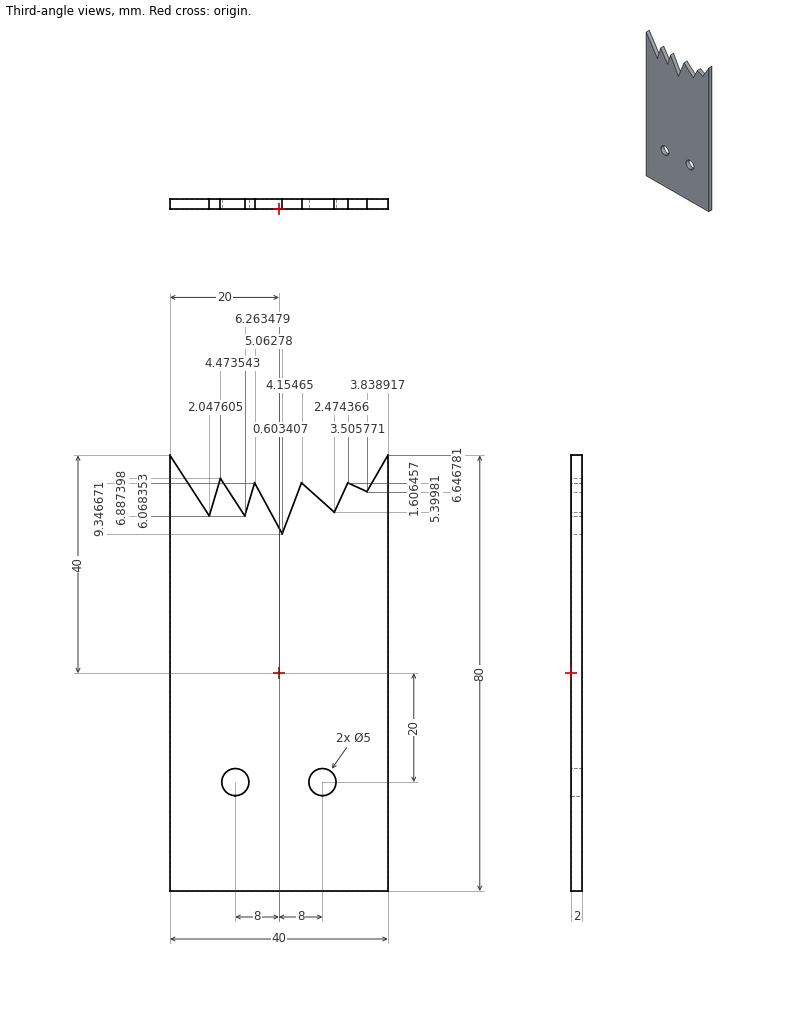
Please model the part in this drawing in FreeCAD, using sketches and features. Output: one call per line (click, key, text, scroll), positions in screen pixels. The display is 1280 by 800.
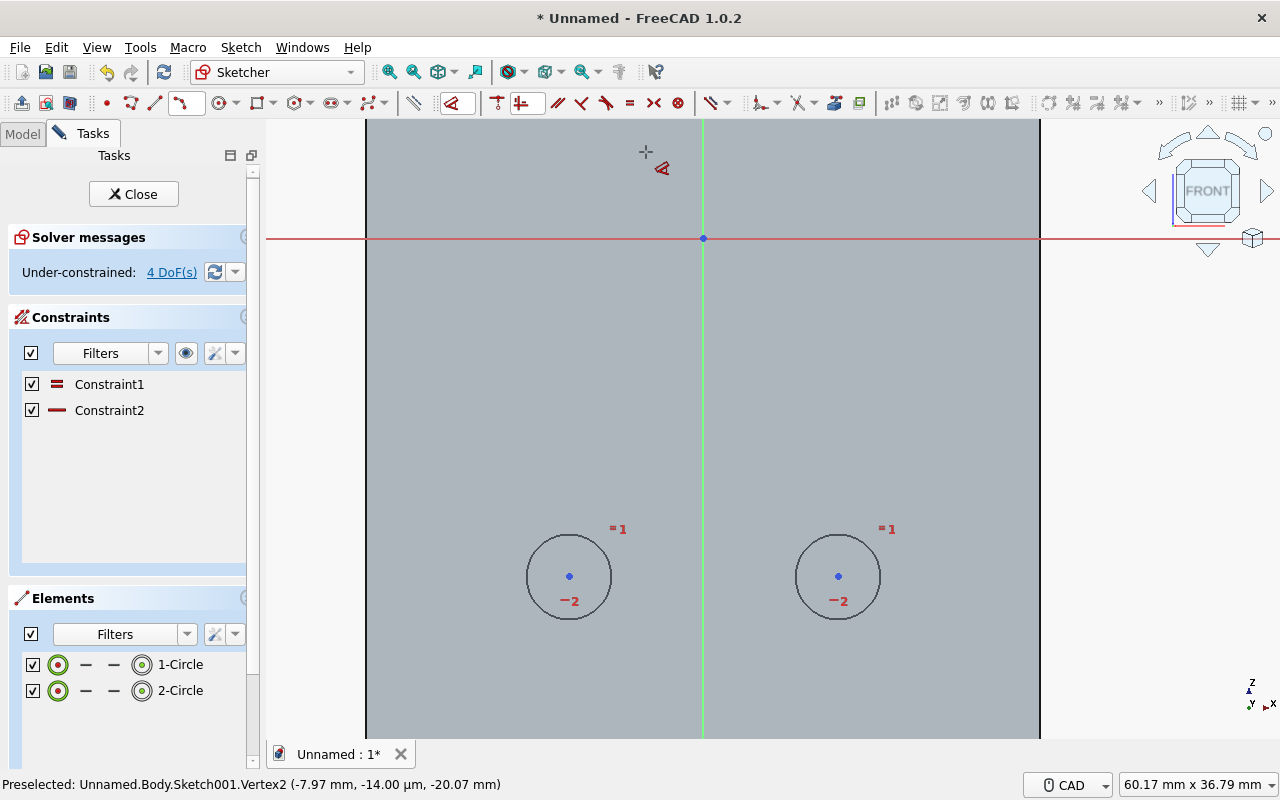
click(868, 547)
click(891, 524)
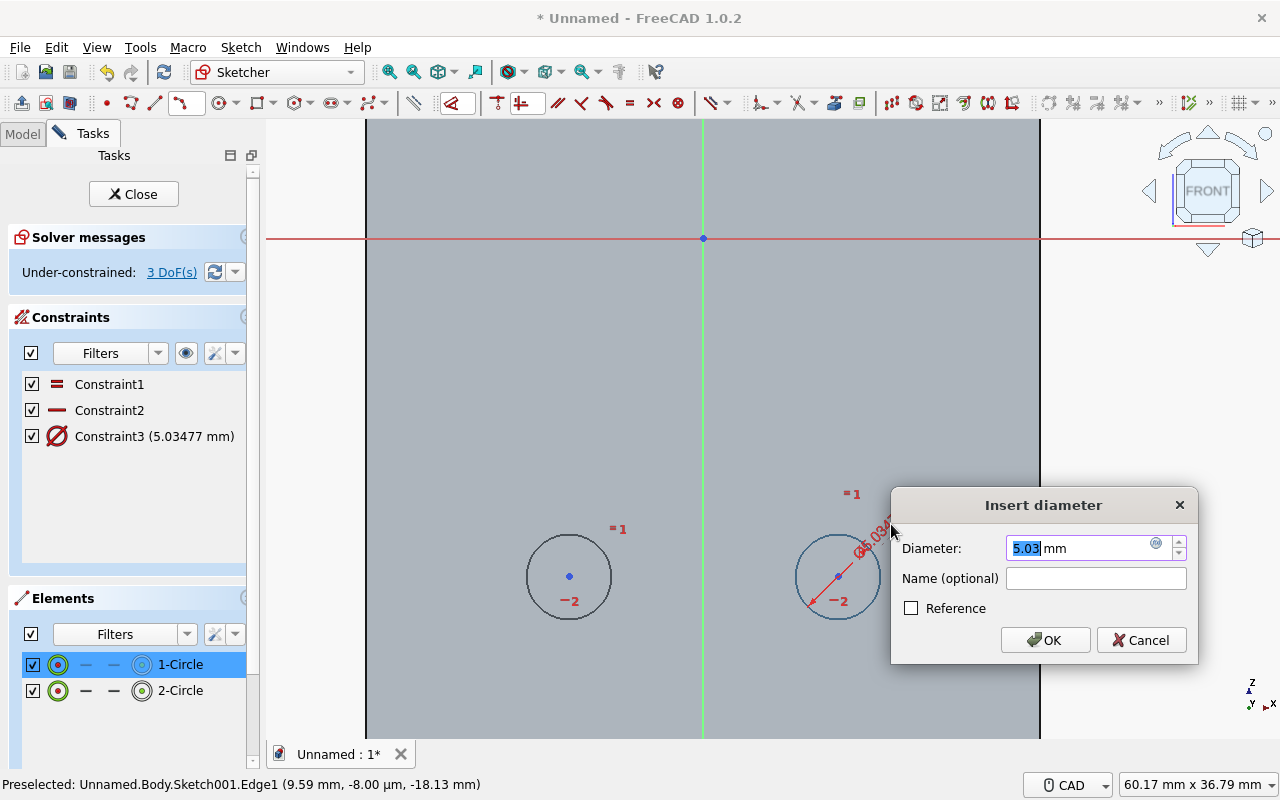
text(5)
key(Return)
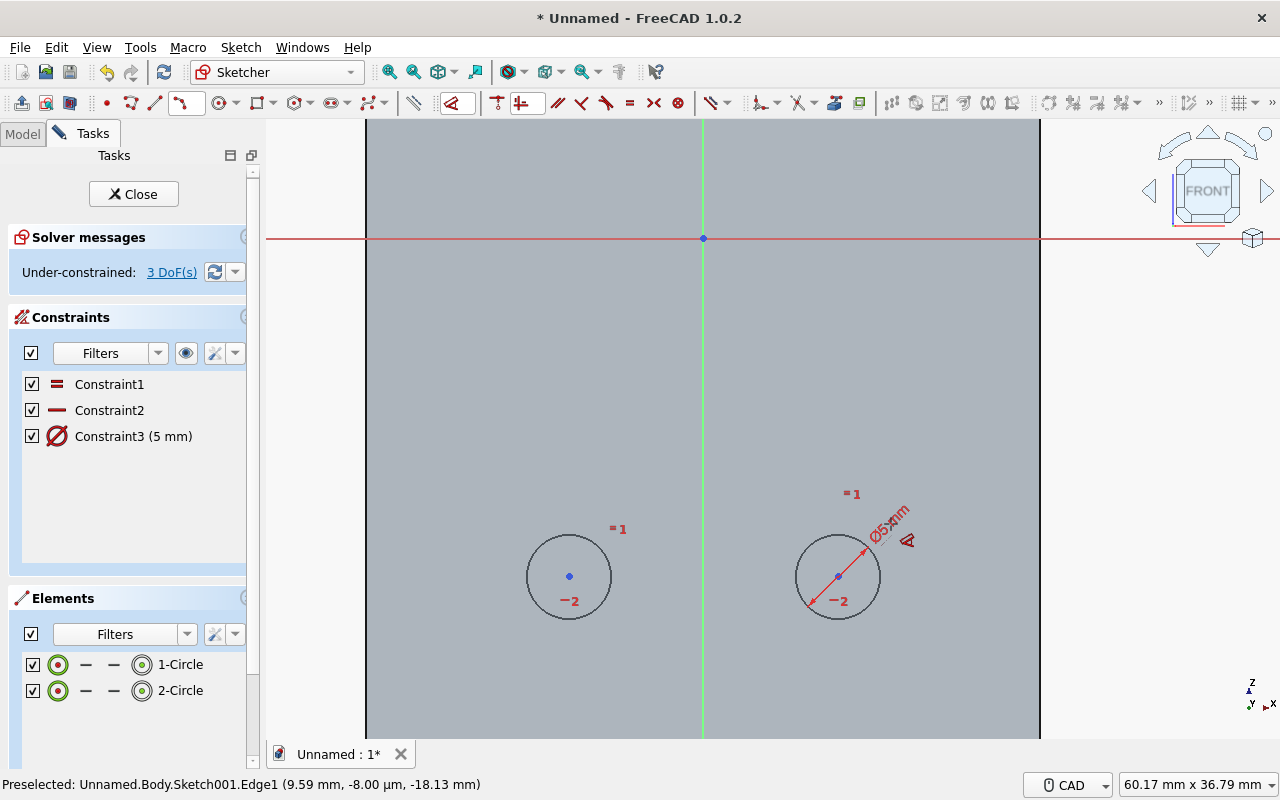
click(838, 577)
click(771, 205)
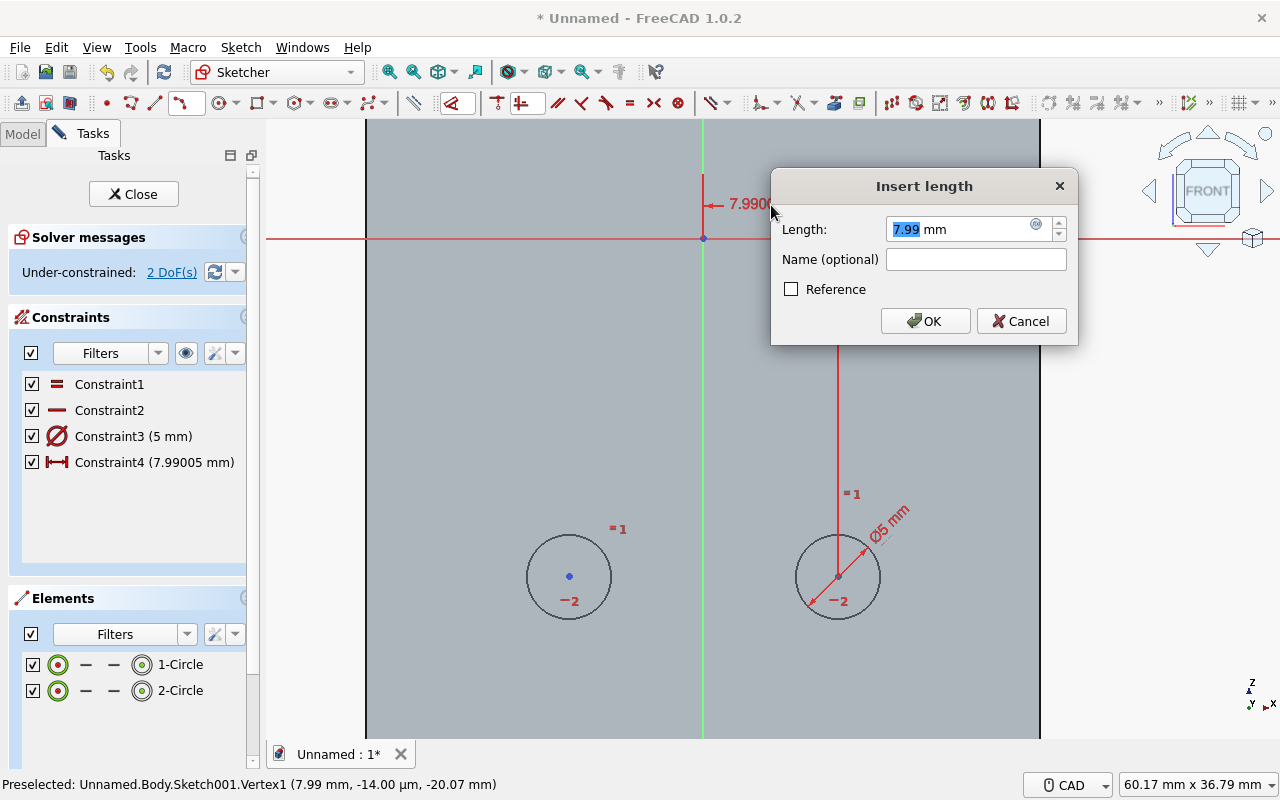
text(8)
key(Return)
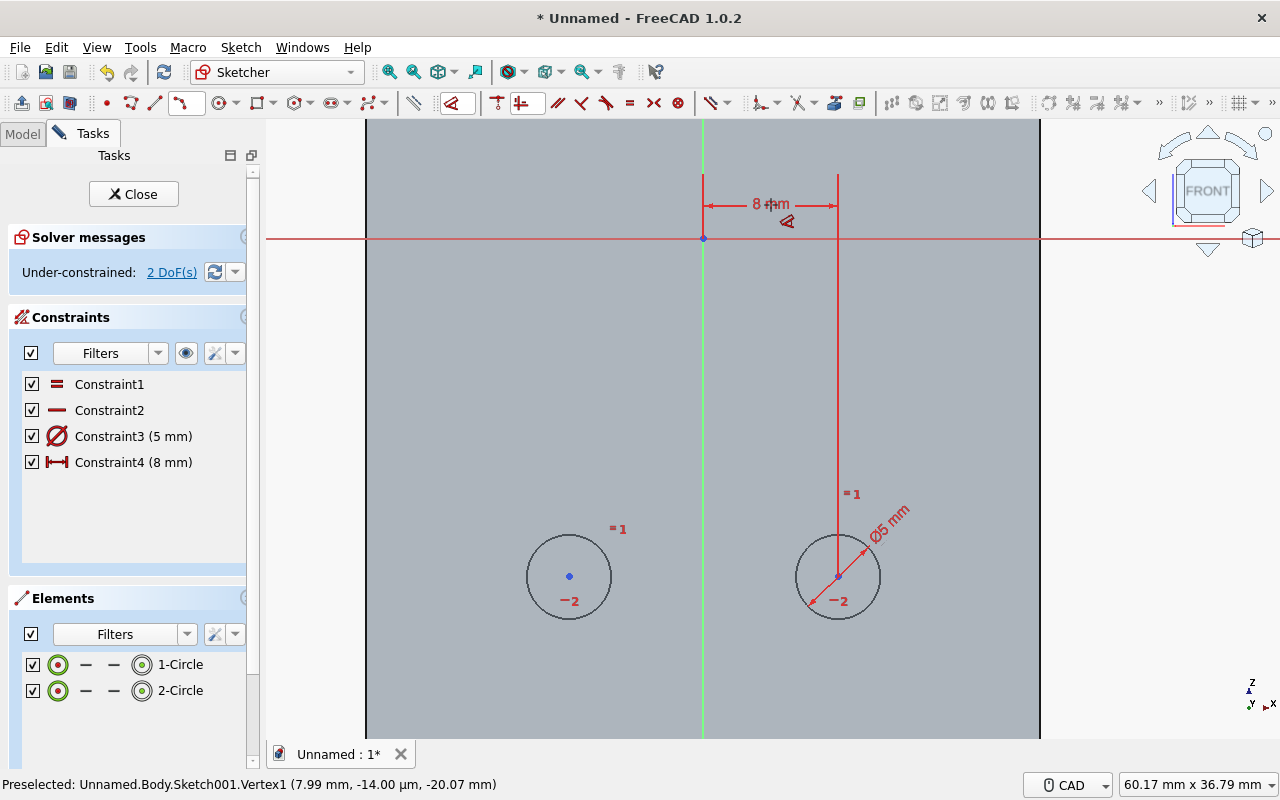
click(569, 577)
click(636, 205)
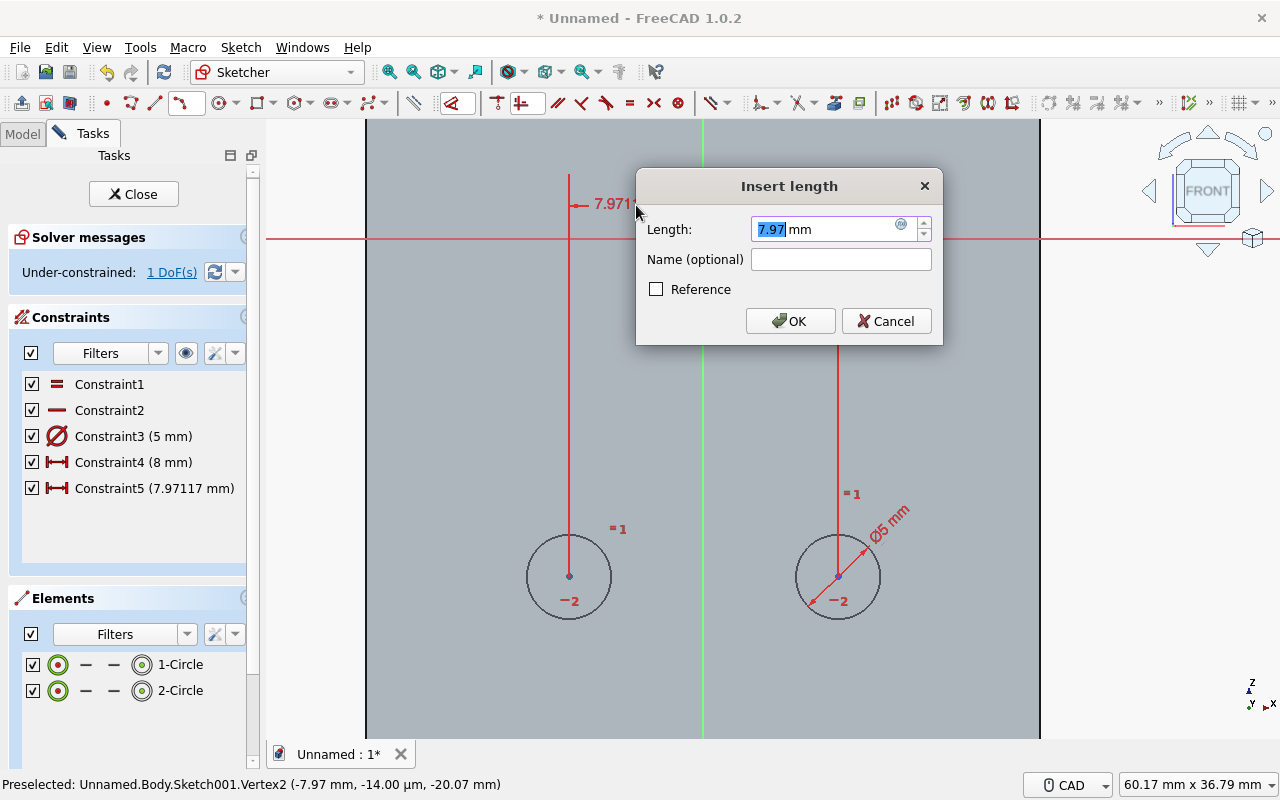
text(8)
key(Return)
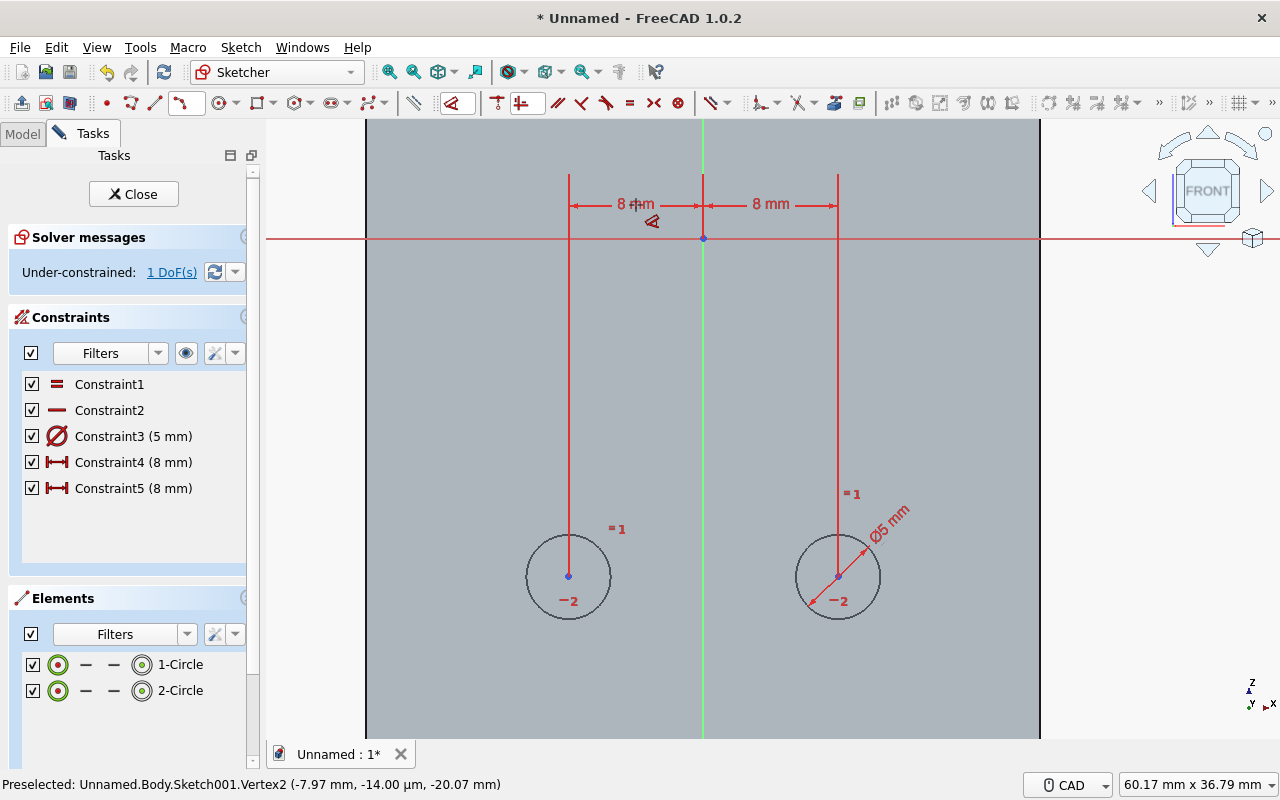
click(838, 577)
click(872, 408)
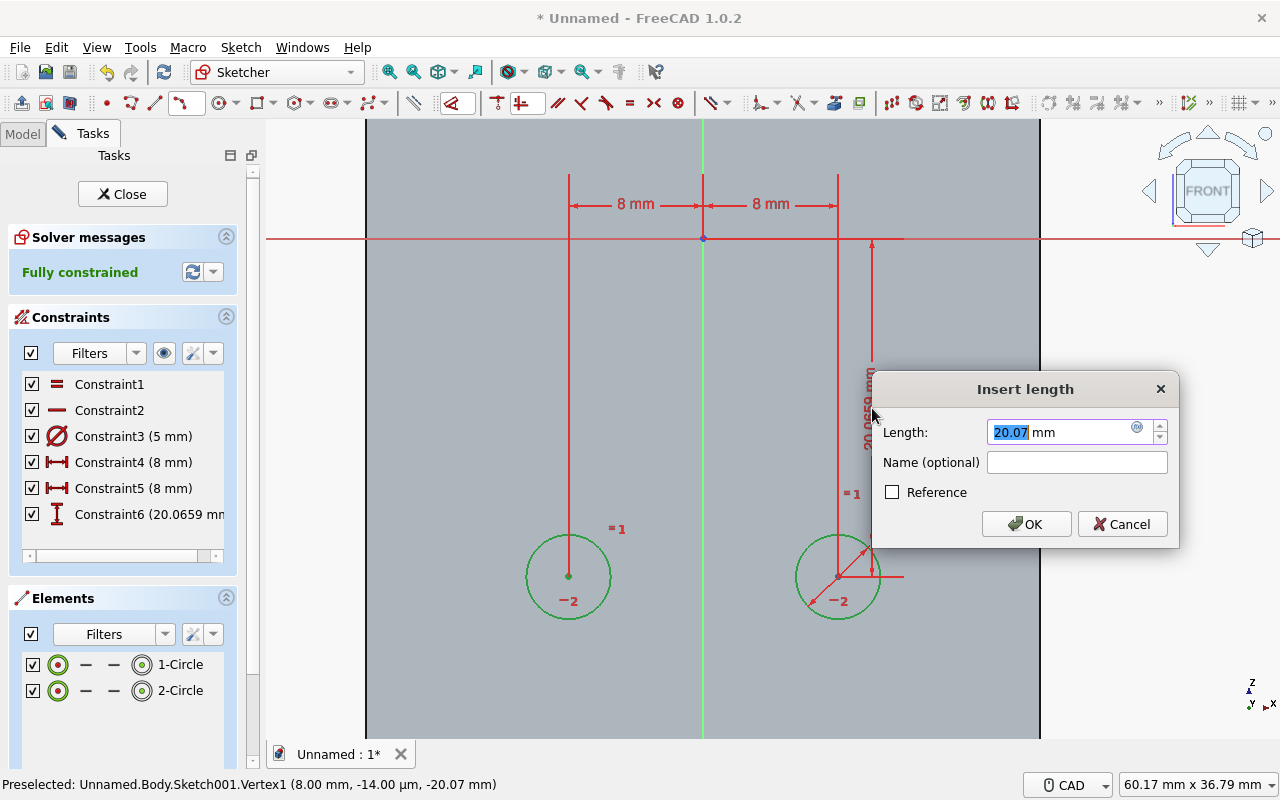
text(20)
key(Return)
key(Escape)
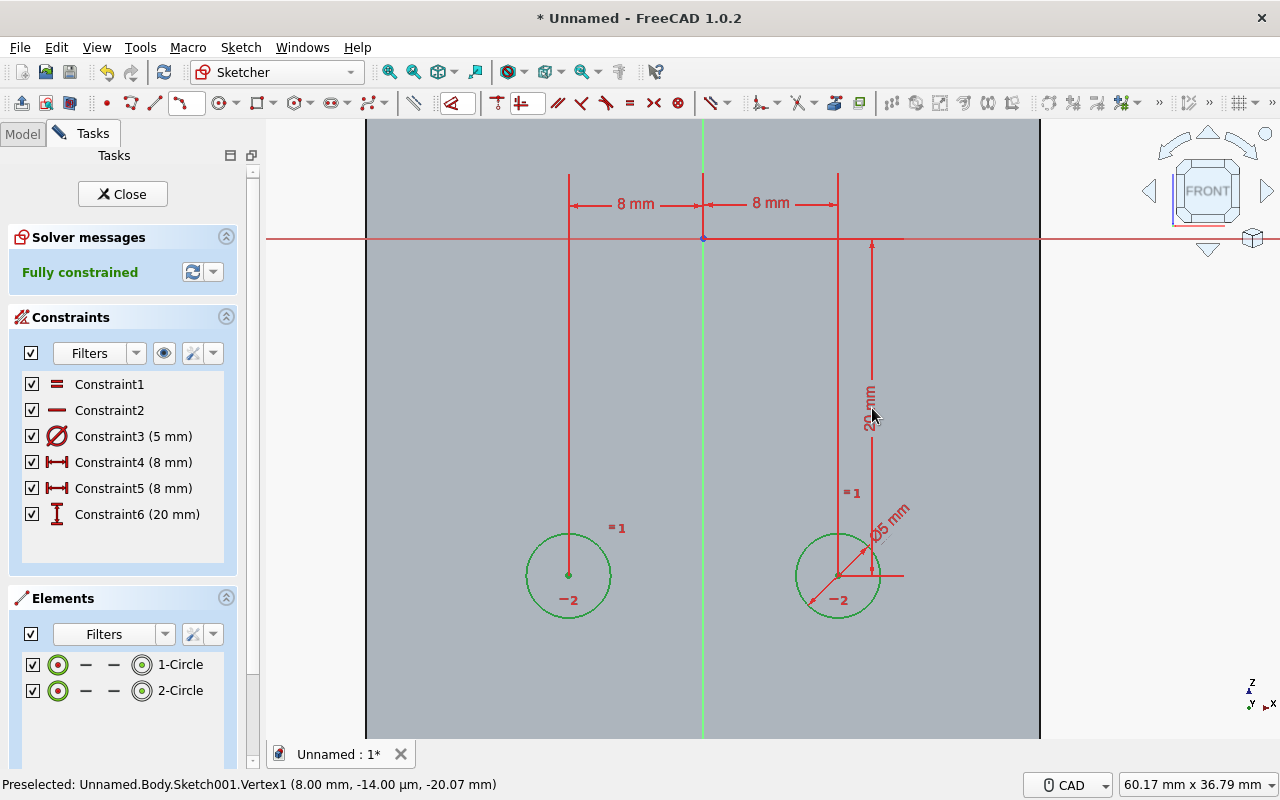
click(123, 194)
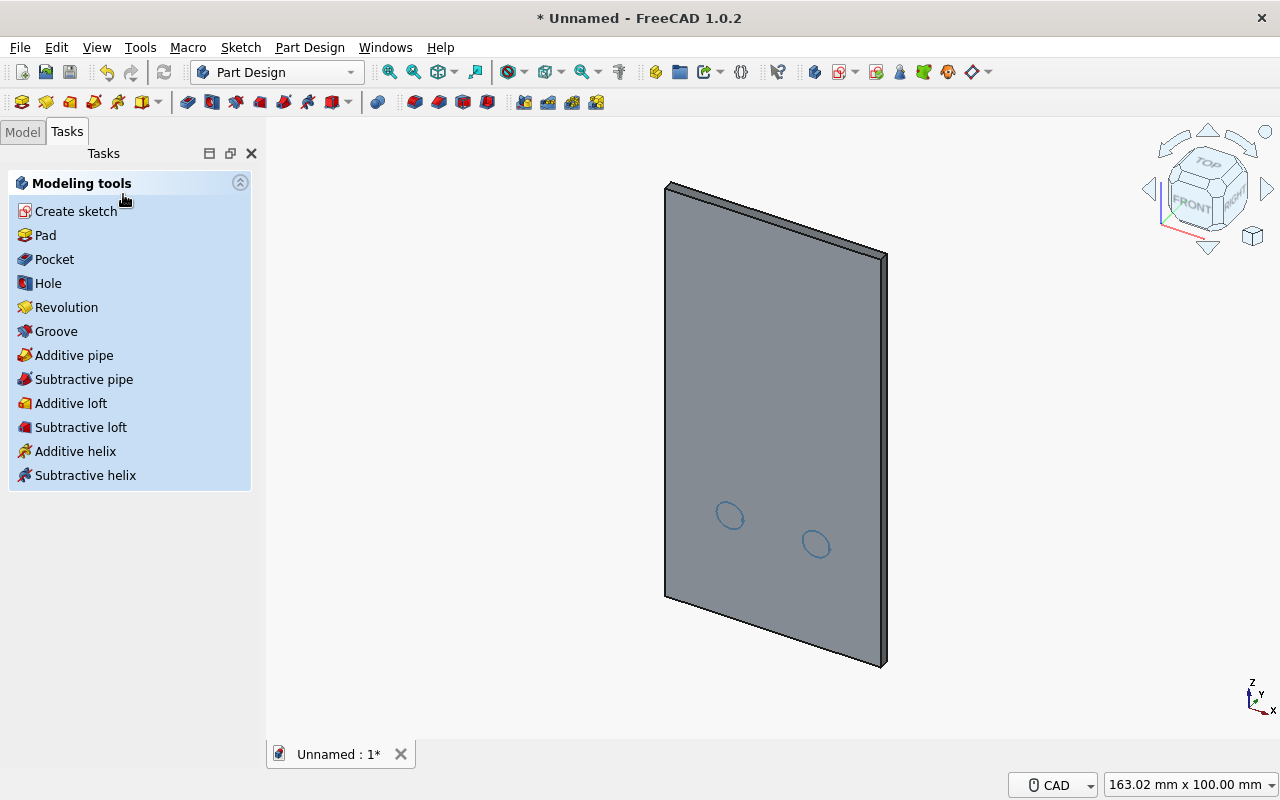
click(188, 102)